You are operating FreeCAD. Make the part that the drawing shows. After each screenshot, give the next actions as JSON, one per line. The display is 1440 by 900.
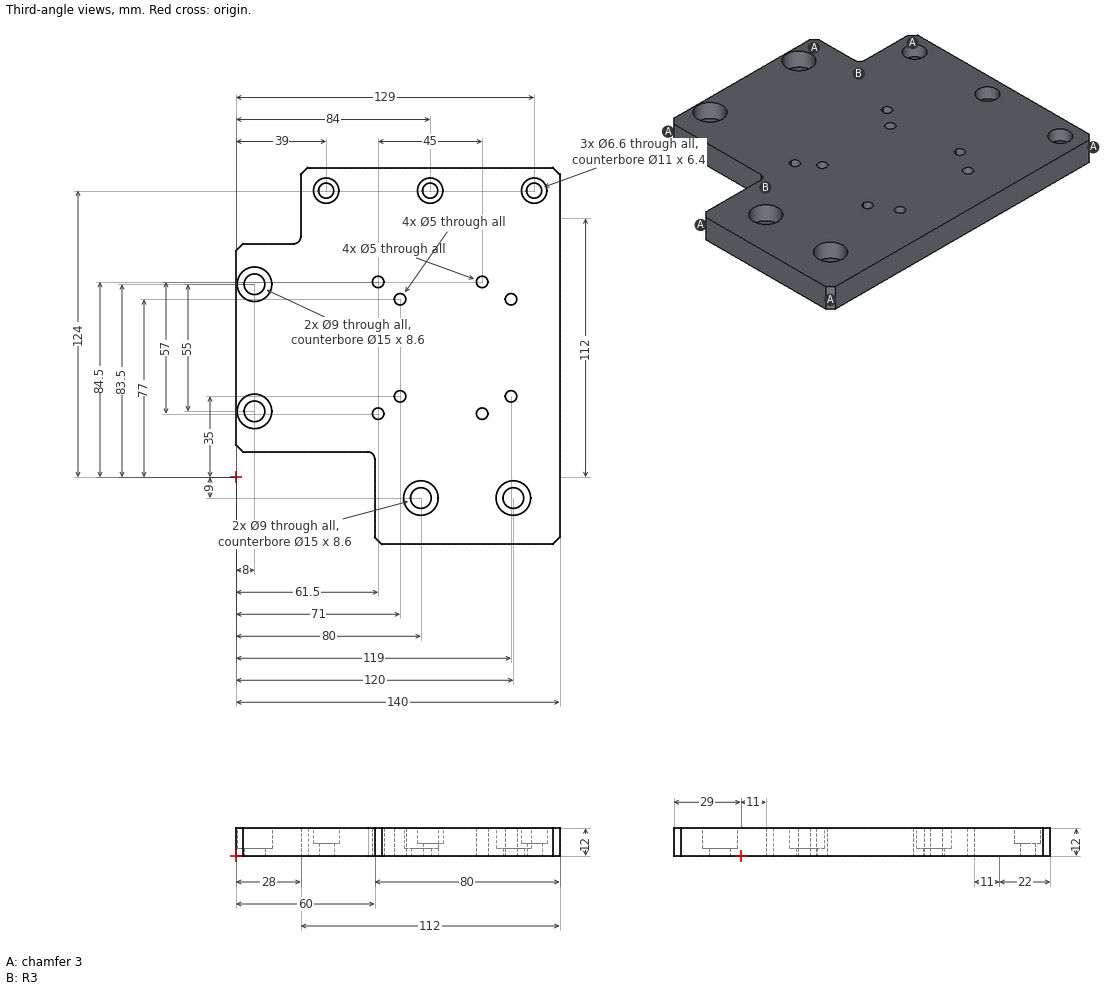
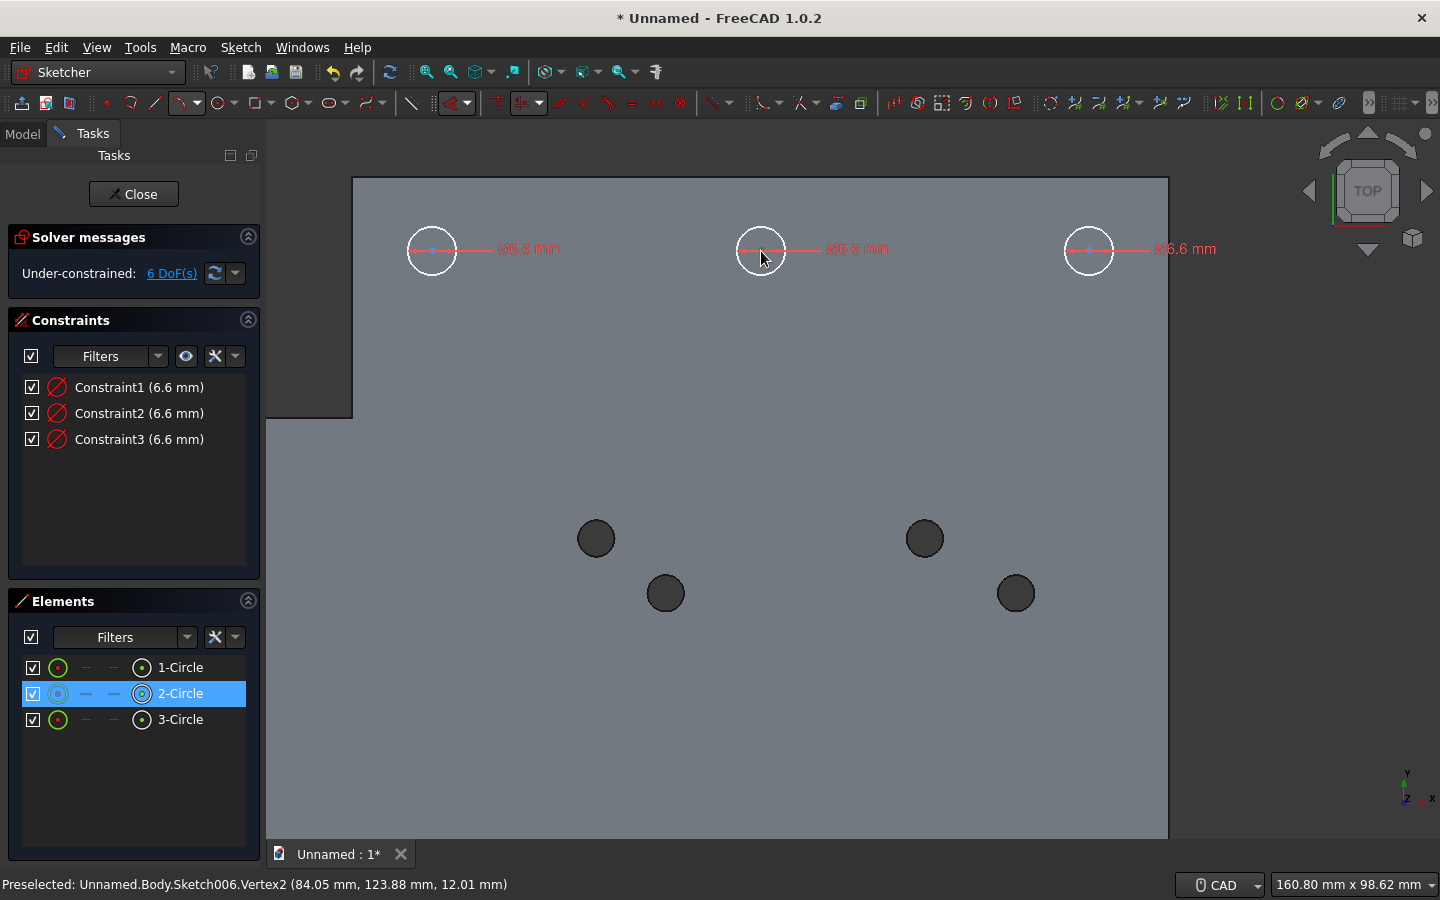
{"action": "left_click", "coordinate": [470, 104]}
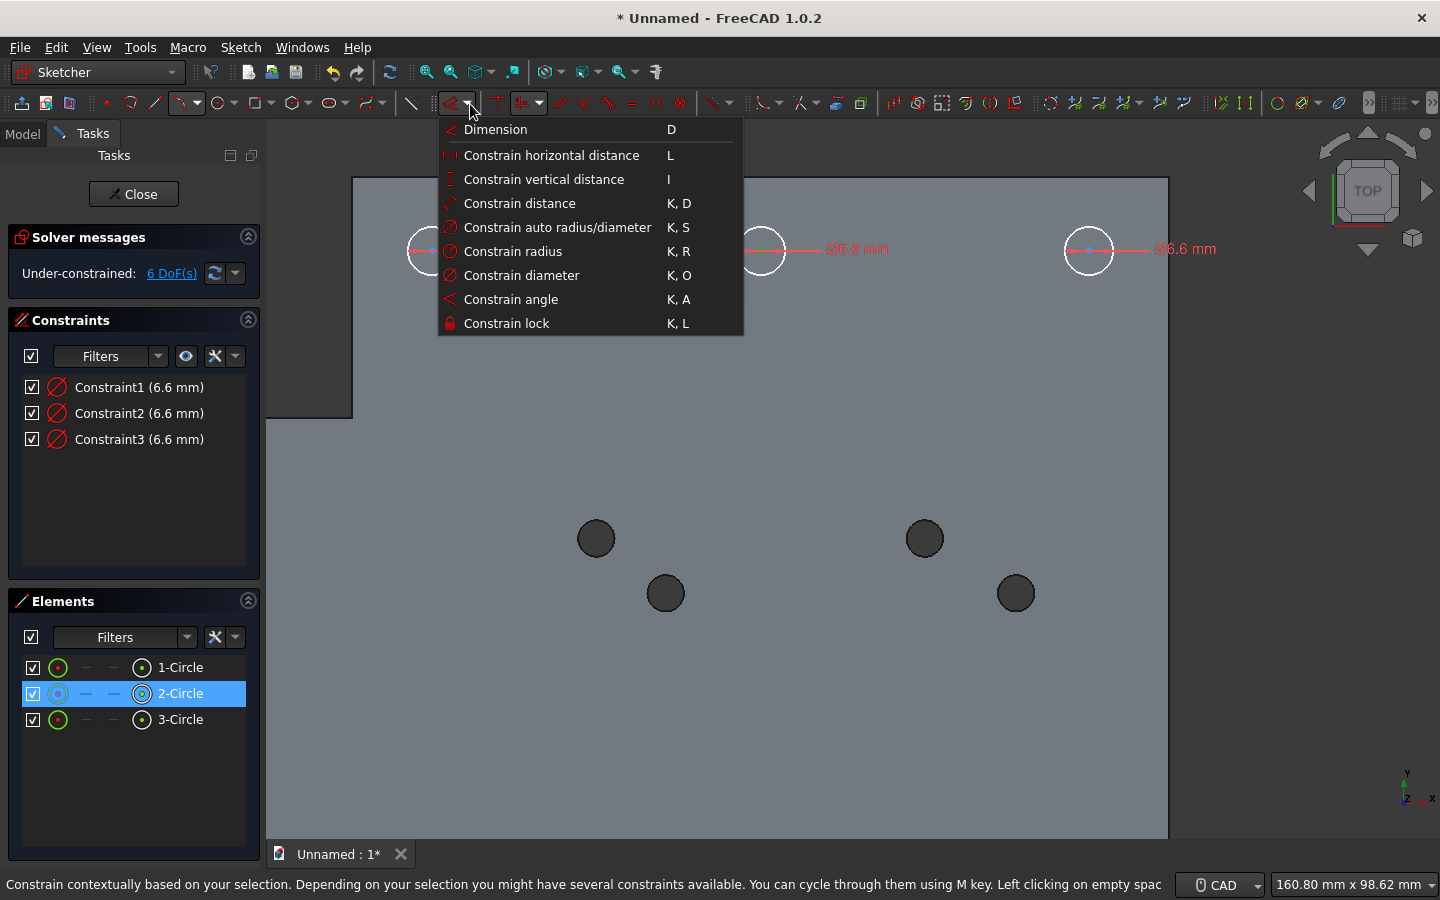
{"action": "left_click", "coordinate": [591, 155]}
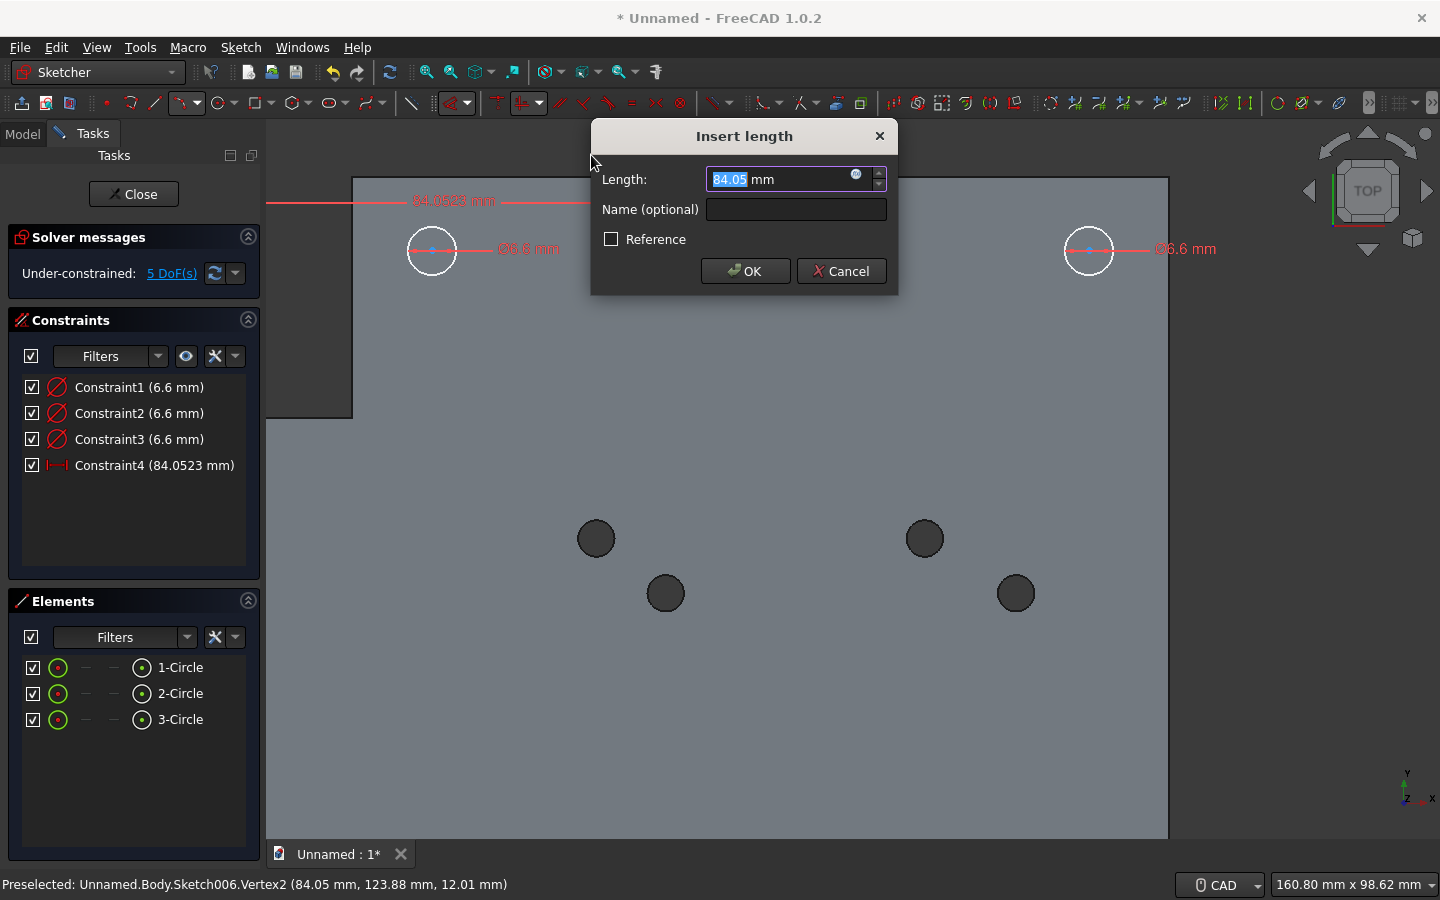
{"action": "type", "text": "84"}
{"action": "key", "text": "Return"}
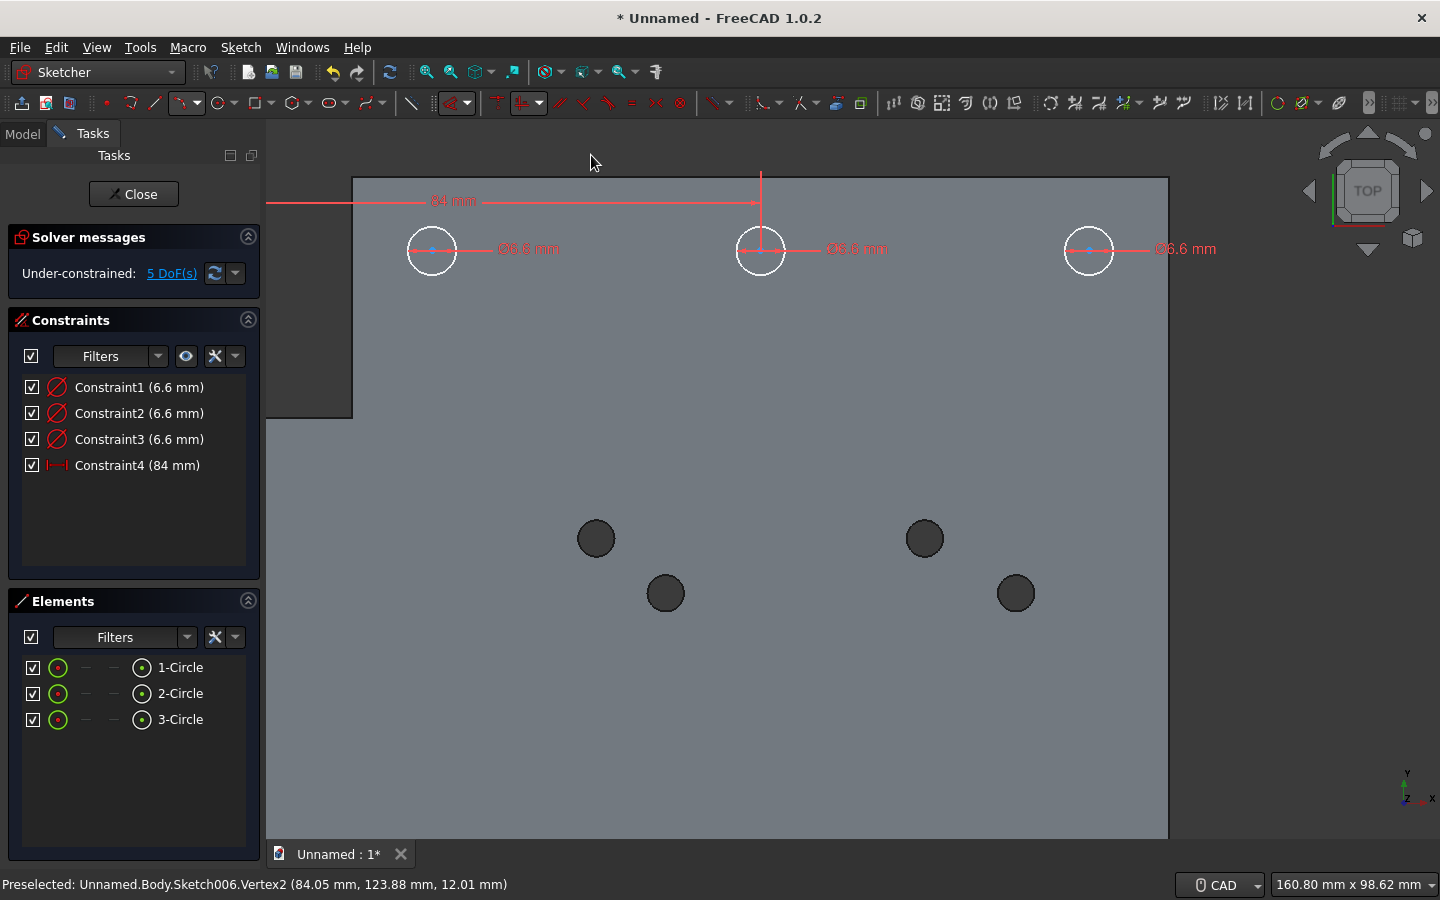
{"action": "left_click", "coordinate": [432, 251]}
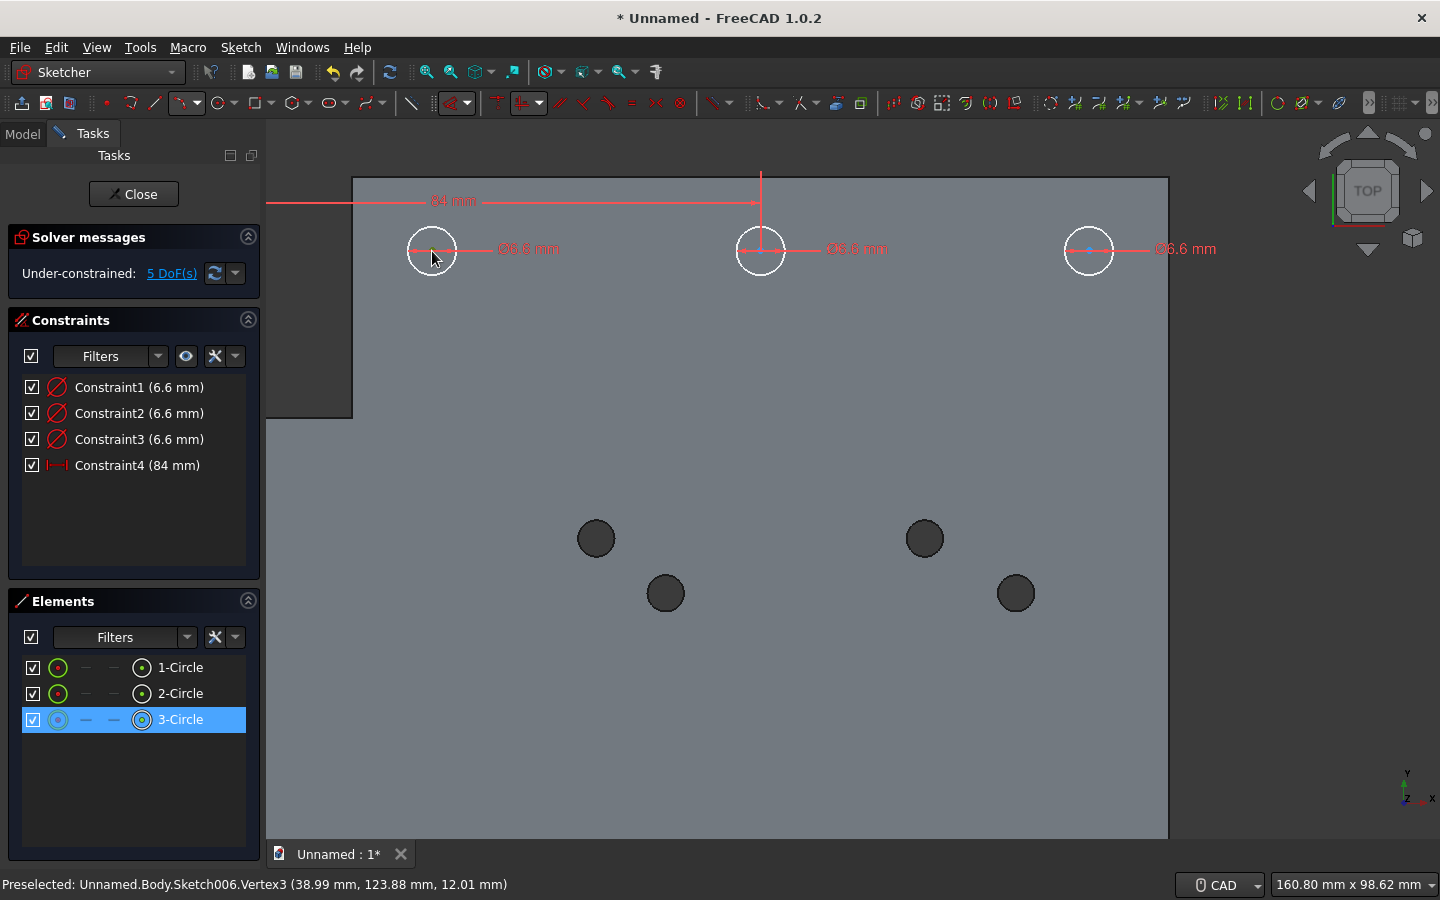
{"action": "left_click", "coordinate": [470, 104]}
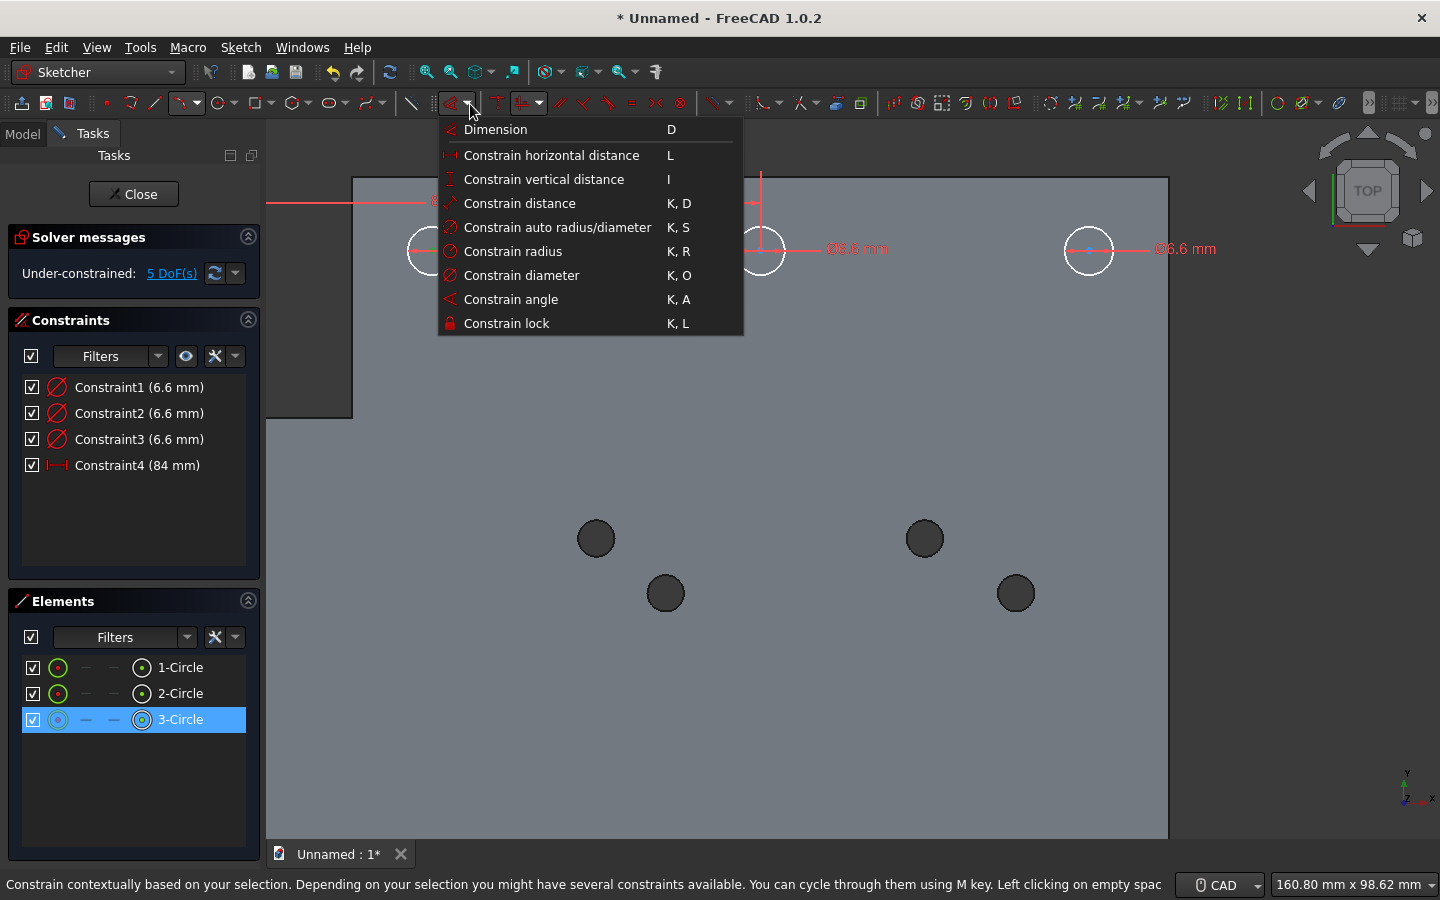
{"action": "left_click", "coordinate": [591, 155]}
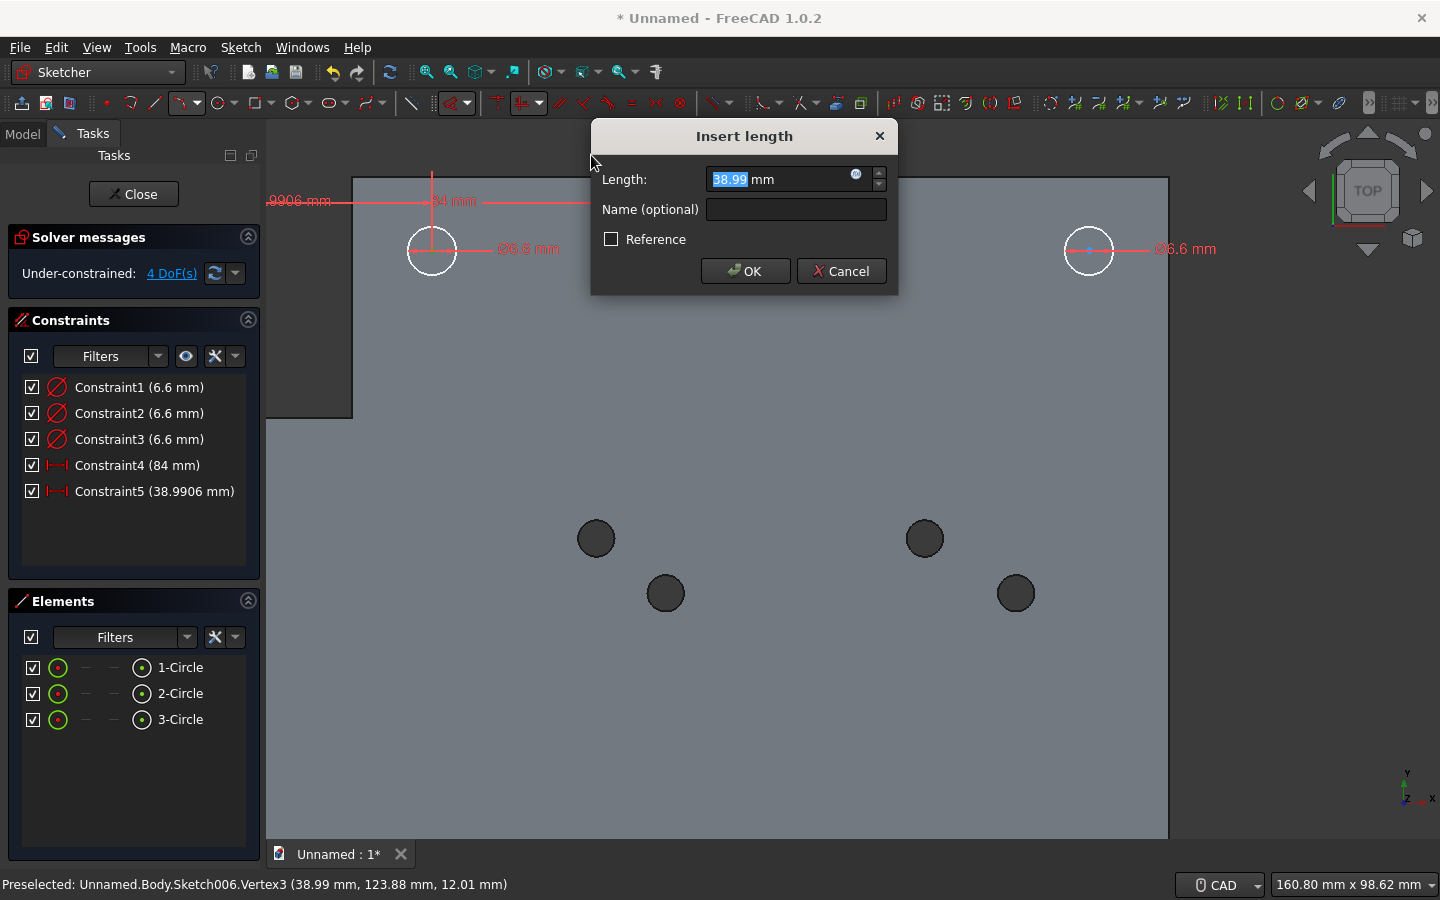
{"action": "type", "text": "39"}
{"action": "key", "text": "Return"}